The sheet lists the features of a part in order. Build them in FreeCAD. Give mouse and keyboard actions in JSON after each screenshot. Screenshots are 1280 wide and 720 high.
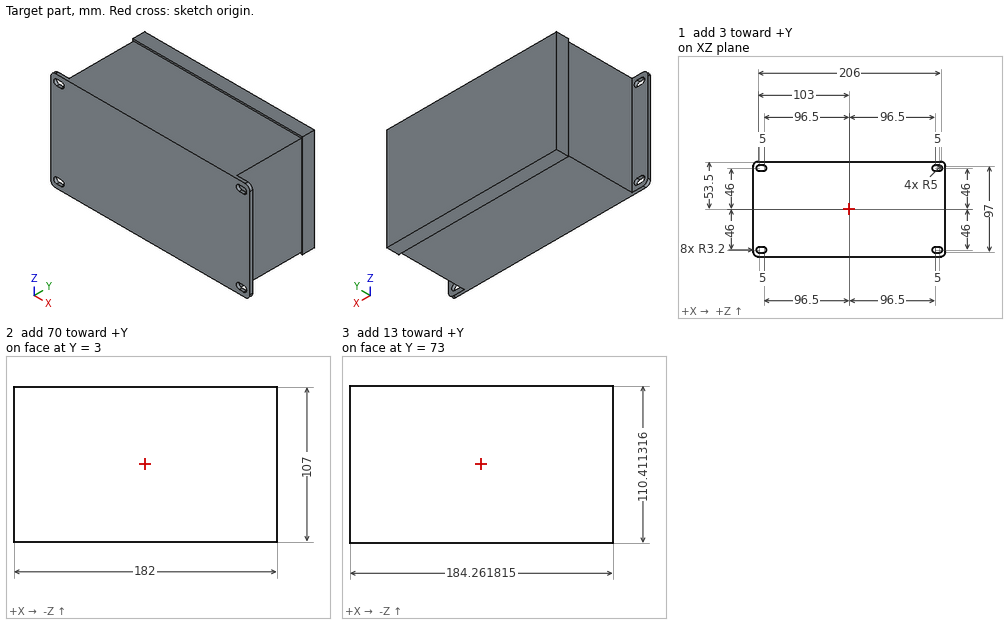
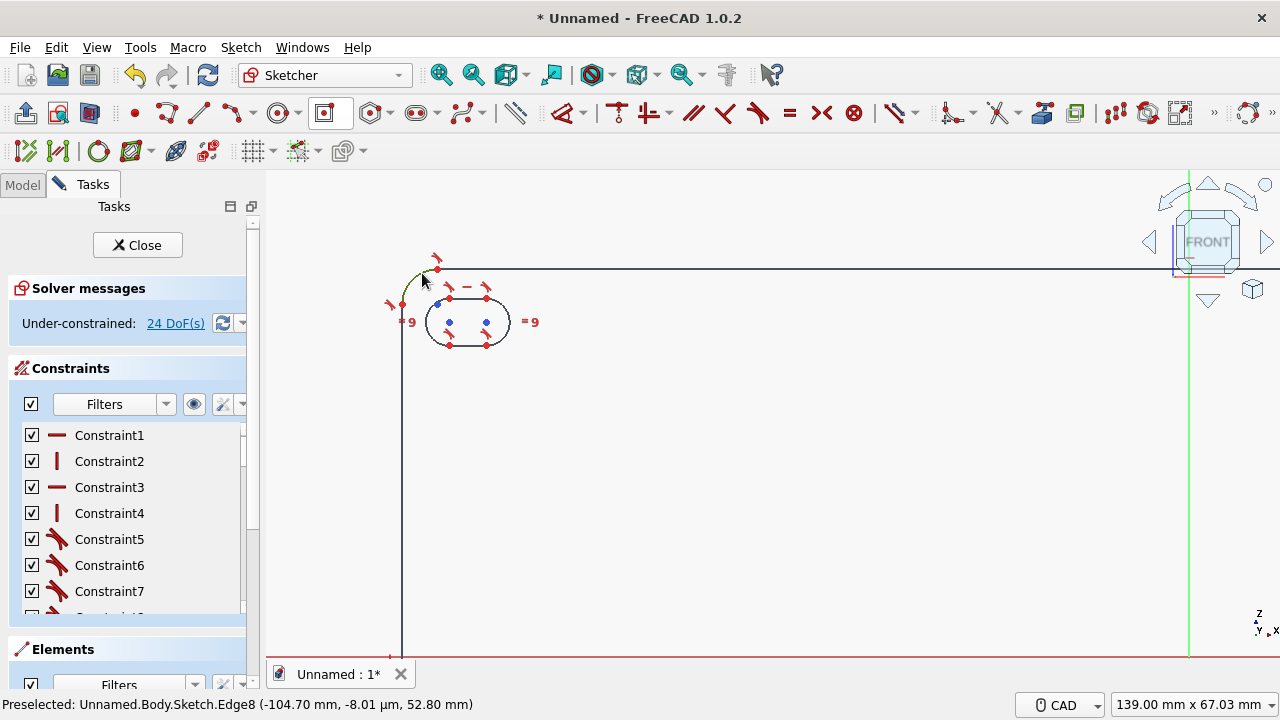
{"action": "left_click", "coordinate": [790, 114]}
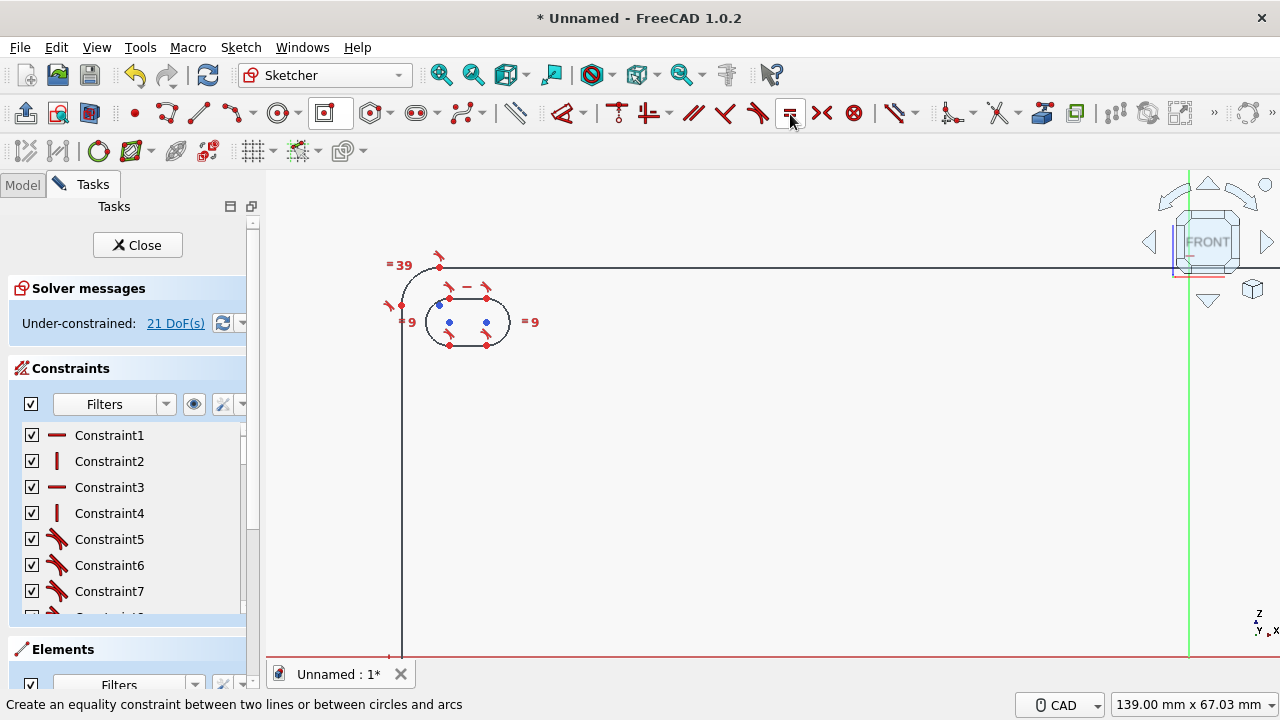
{"action": "left_click", "coordinate": [430, 308]}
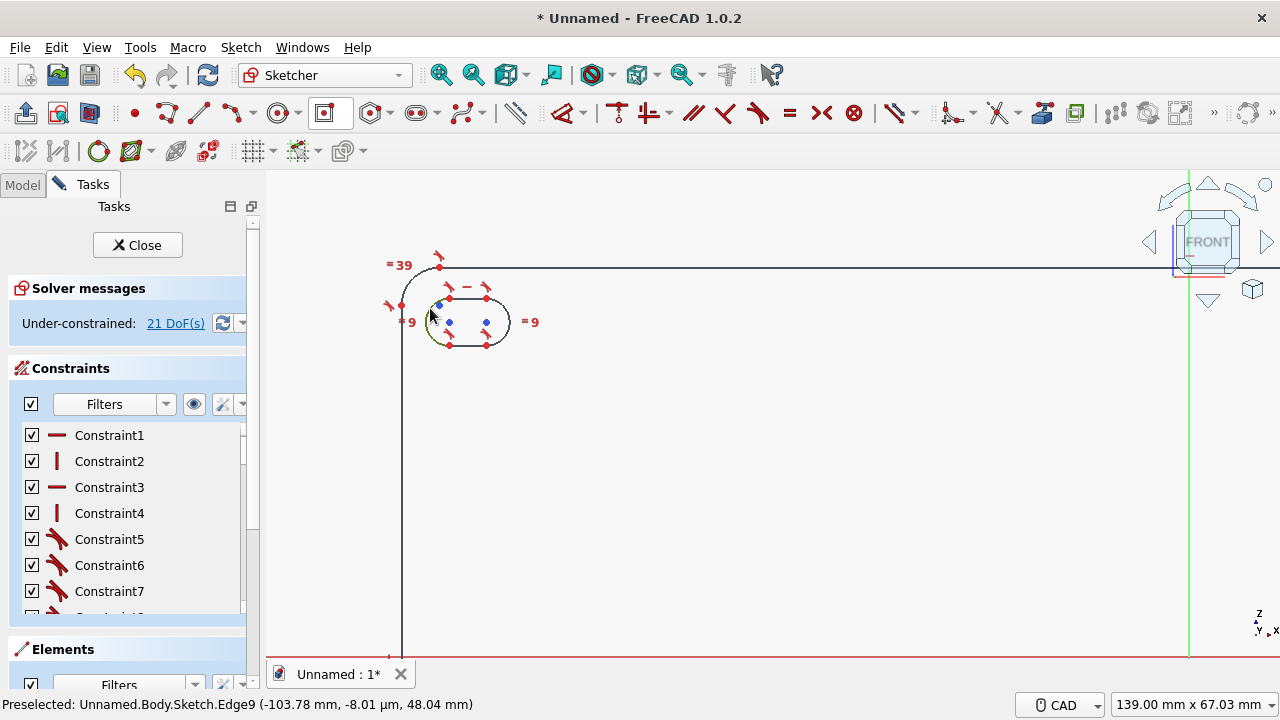
{"action": "scroll", "coordinate": [422, 274], "scroll_direction": "down", "scroll_amount": 5}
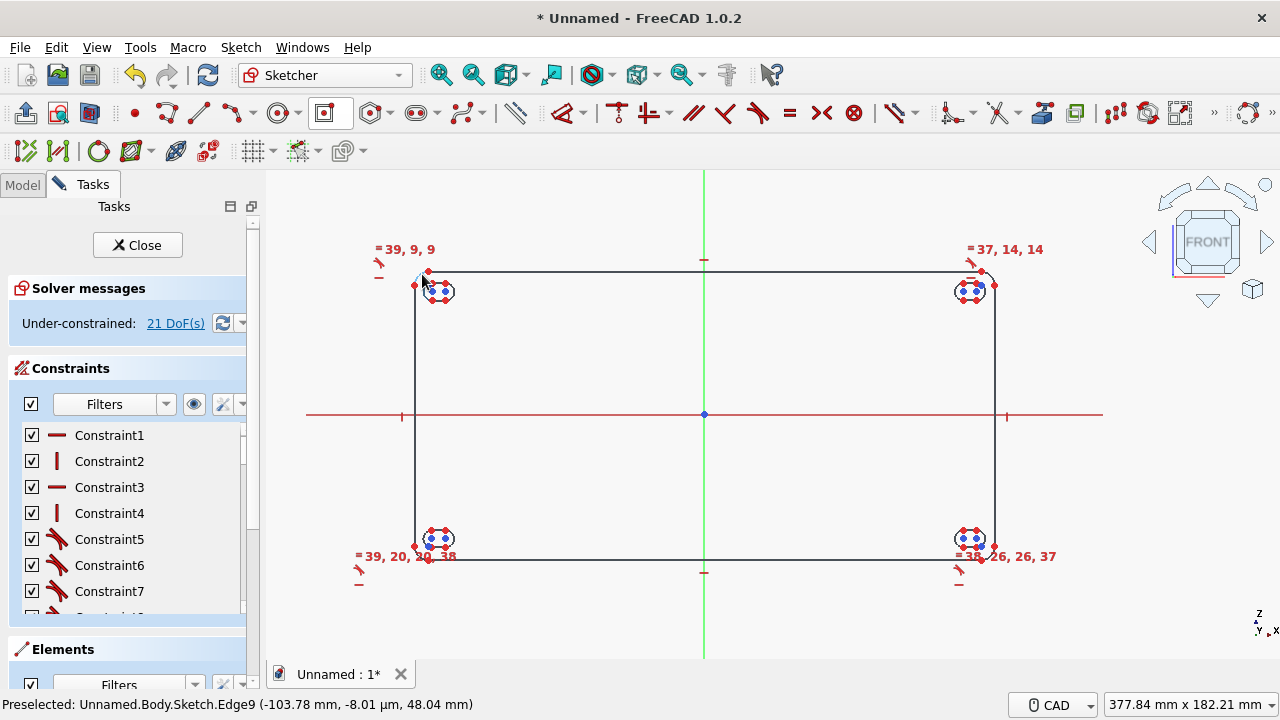
{"action": "scroll", "coordinate": [957, 287], "scroll_direction": "up", "scroll_amount": 3}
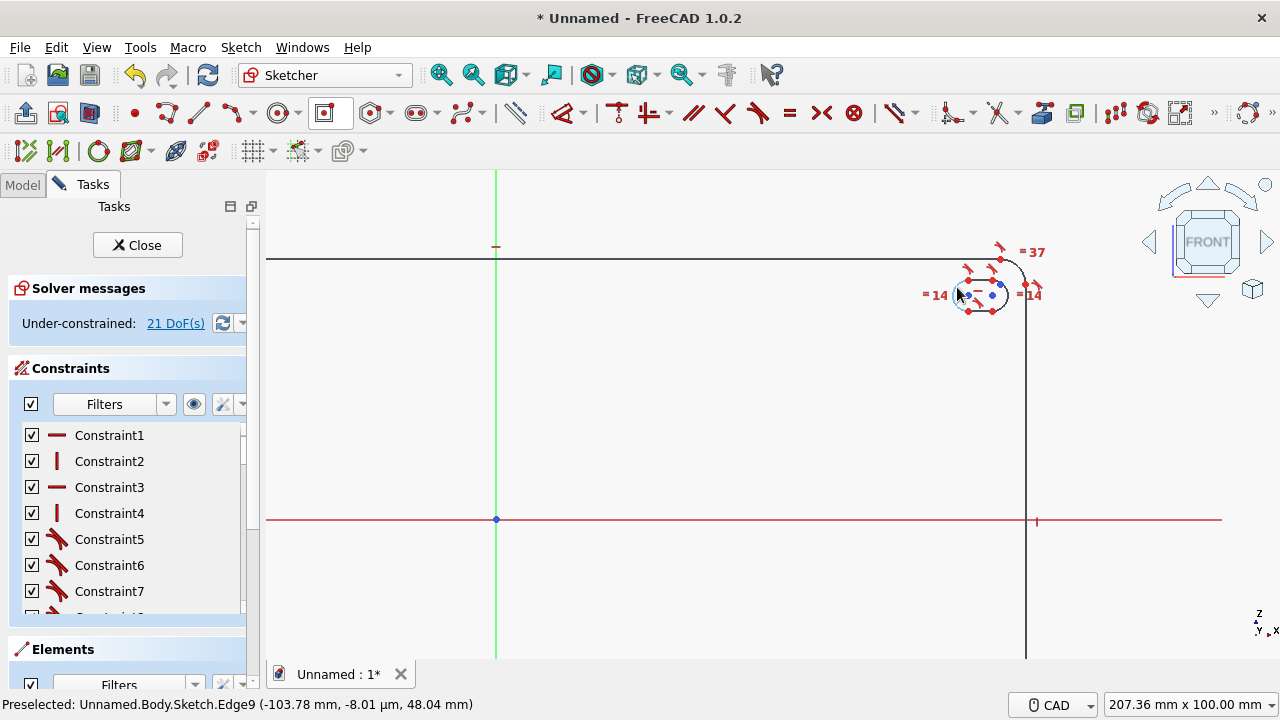
{"action": "left_click", "coordinate": [956, 287]}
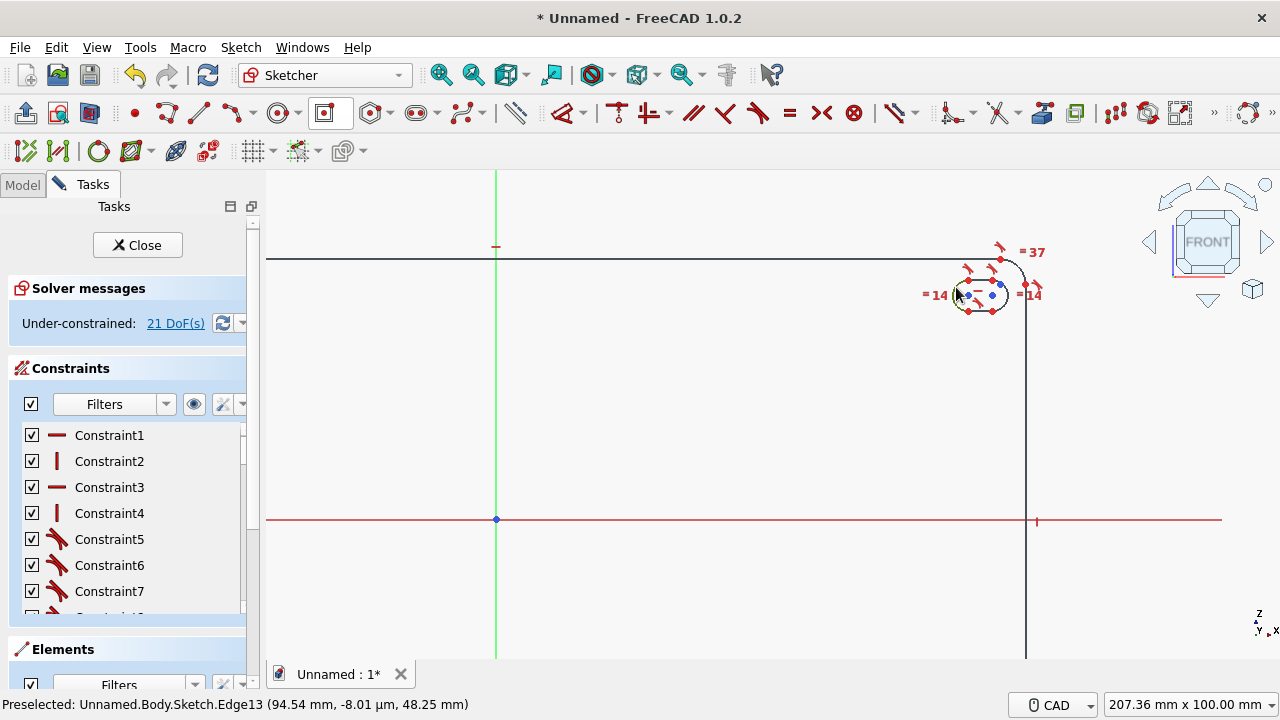
{"action": "scroll", "coordinate": [958, 286], "scroll_direction": "down", "scroll_amount": 3}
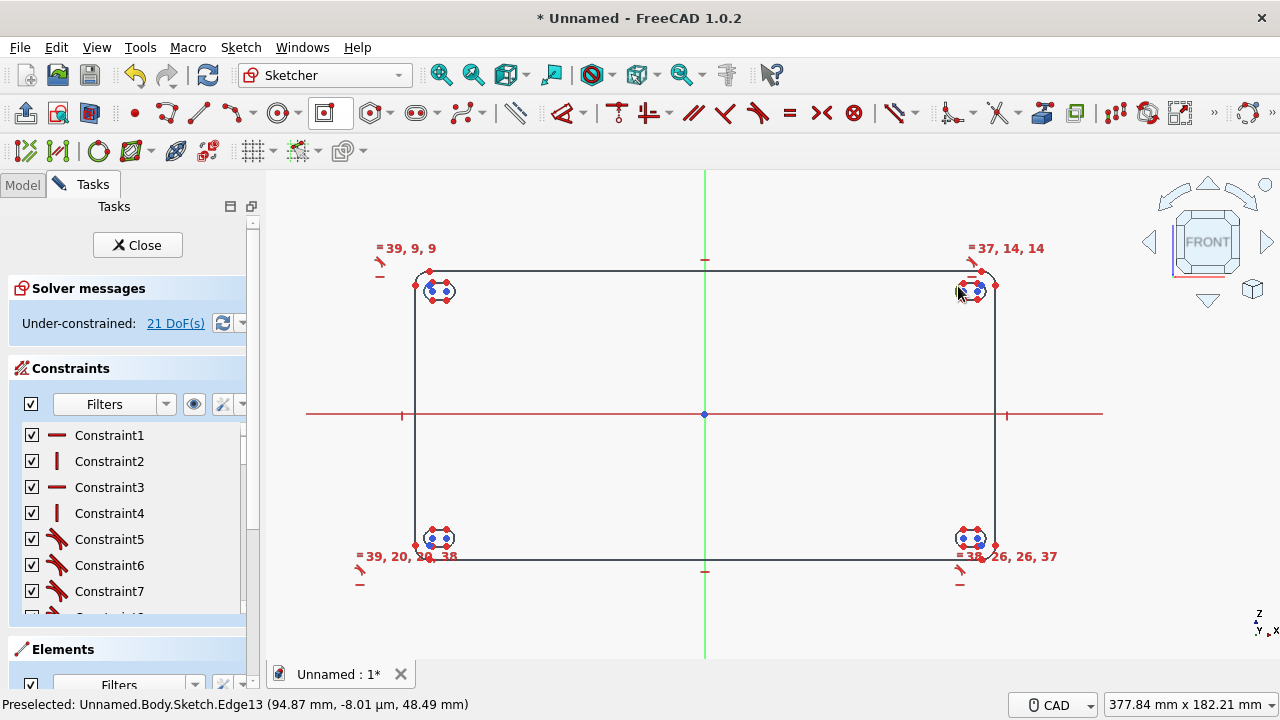
{"action": "scroll", "coordinate": [426, 533], "scroll_direction": "up", "scroll_amount": 3}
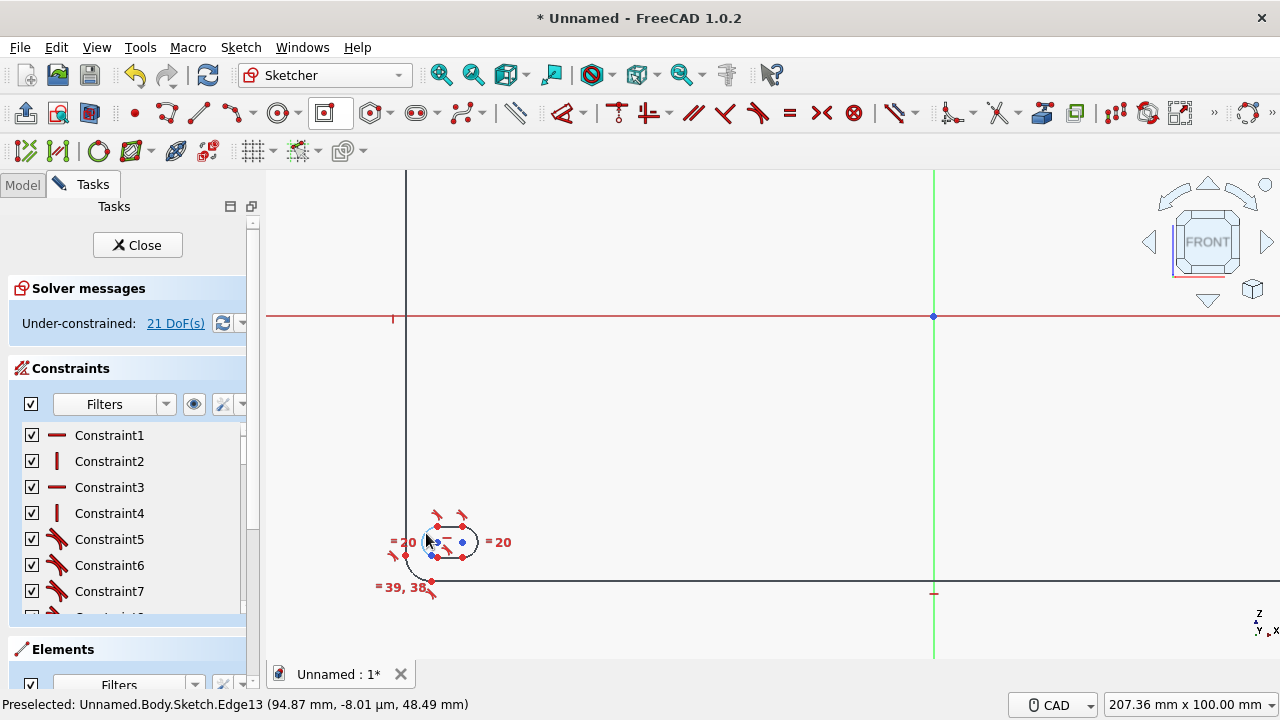
{"action": "left_click", "coordinate": [425, 533]}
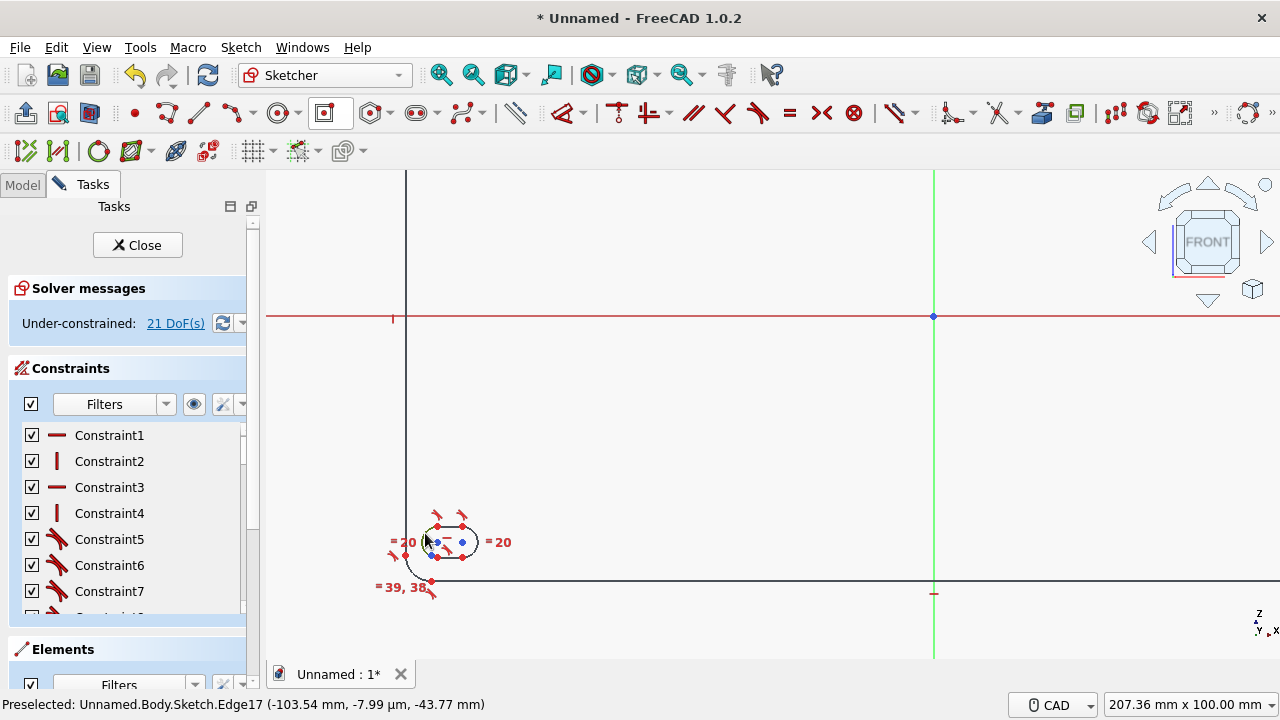
{"action": "scroll", "coordinate": [425, 534], "scroll_direction": "down", "scroll_amount": 3}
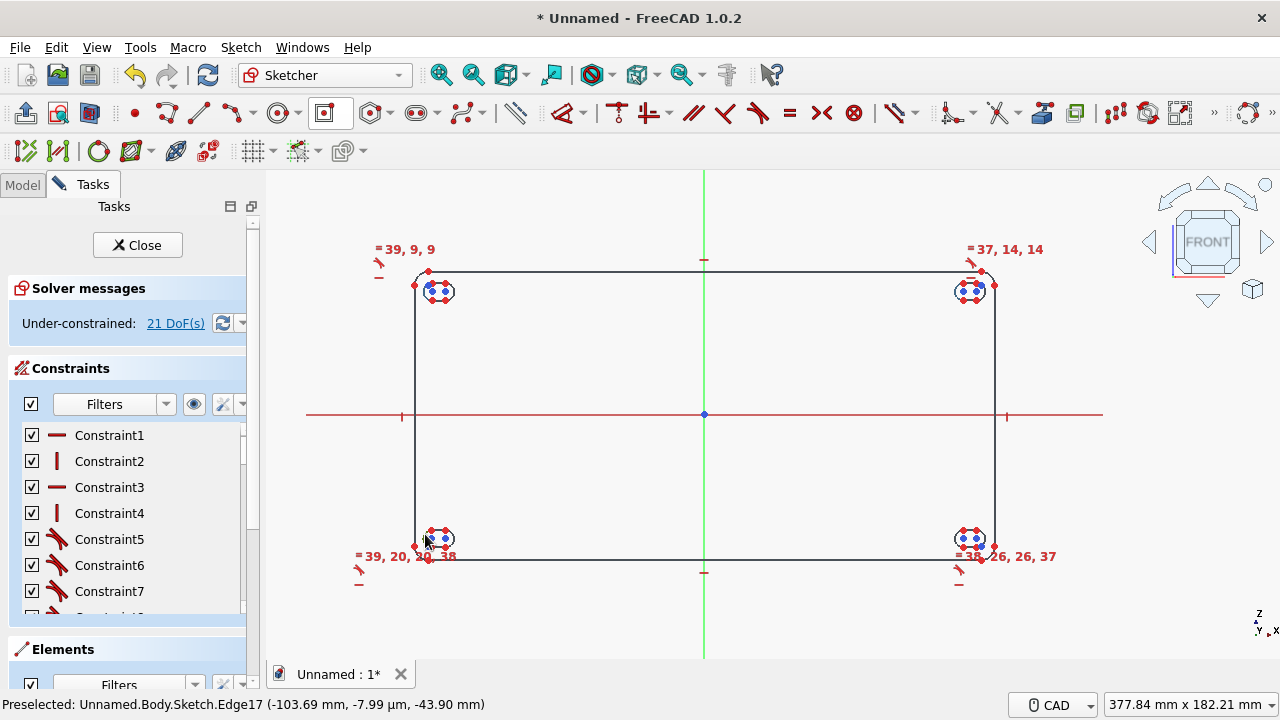
{"action": "scroll", "coordinate": [957, 534], "scroll_direction": "up", "scroll_amount": 3}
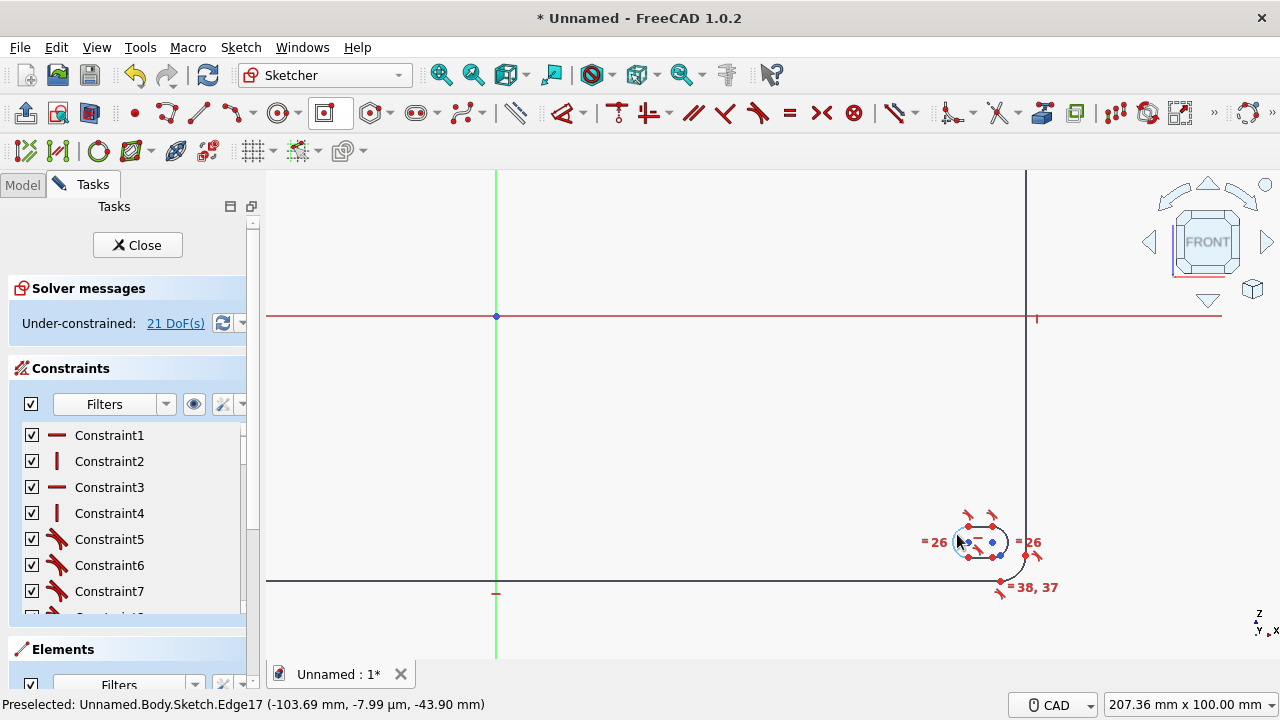
{"action": "left_click", "coordinate": [956, 533]}